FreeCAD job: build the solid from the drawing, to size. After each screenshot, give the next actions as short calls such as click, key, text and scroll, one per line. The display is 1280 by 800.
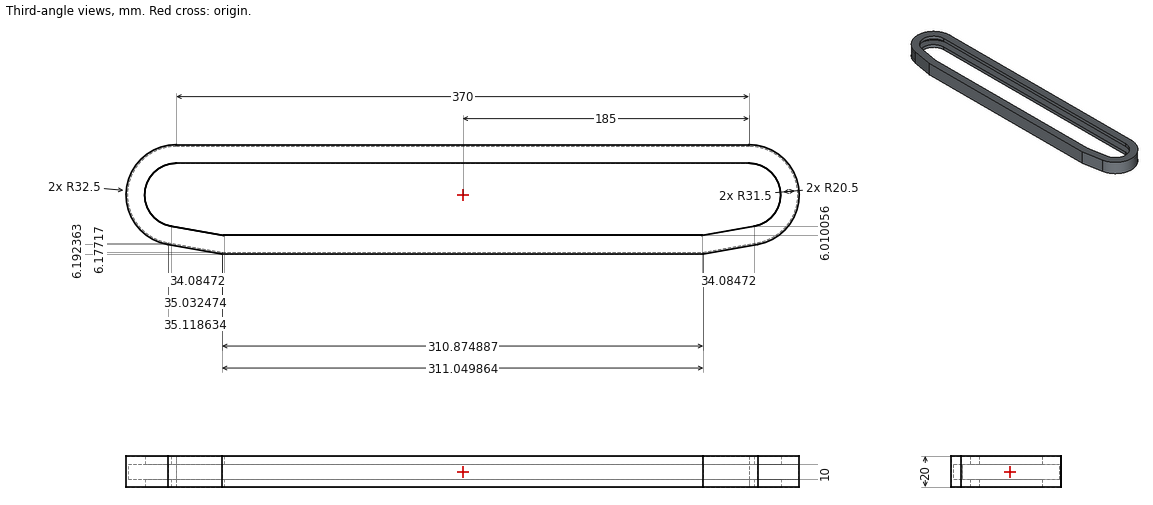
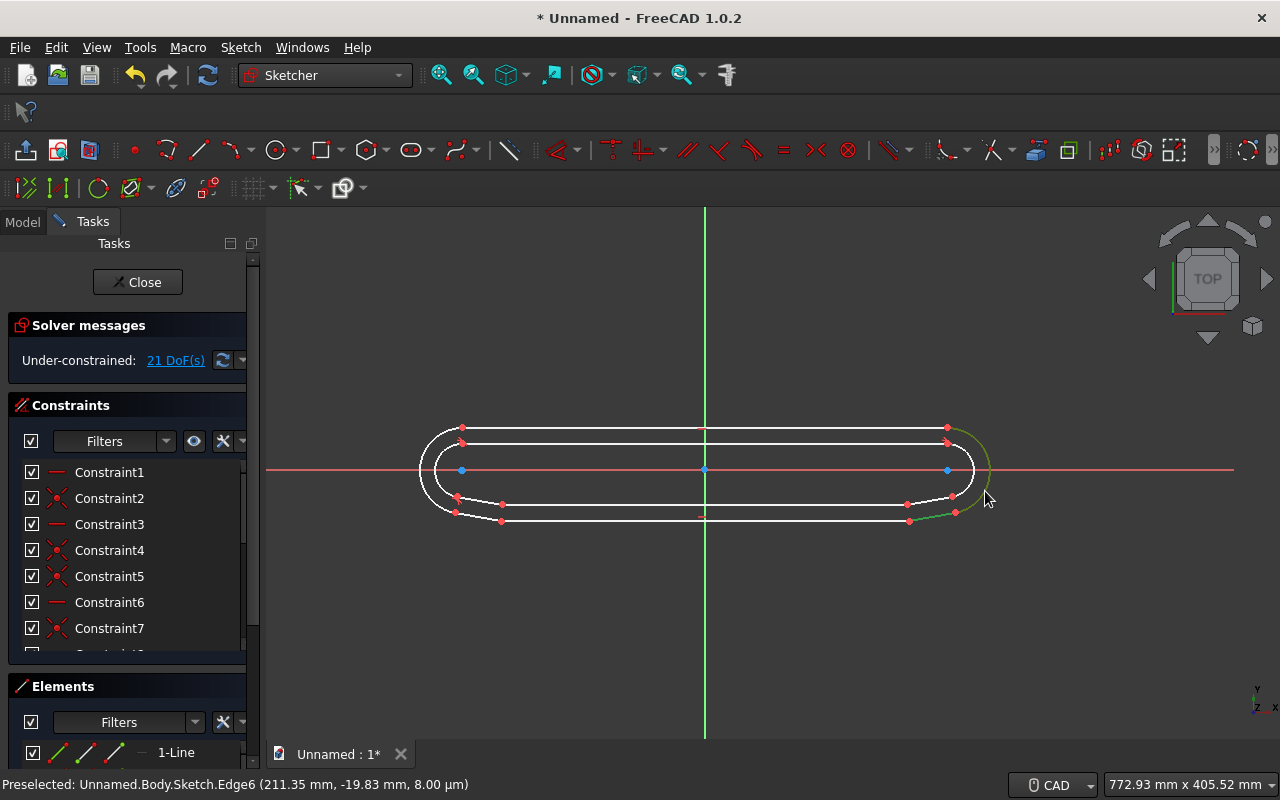
key(t)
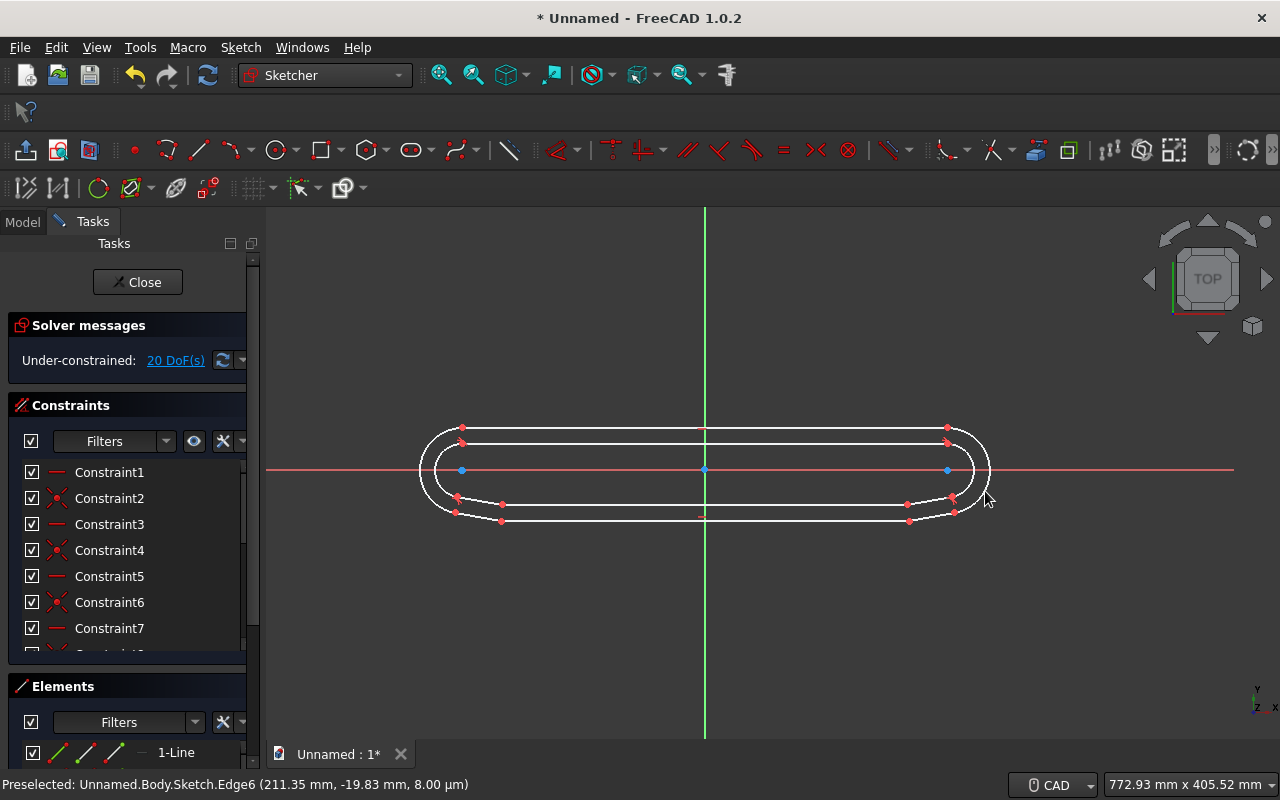
click(607, 444)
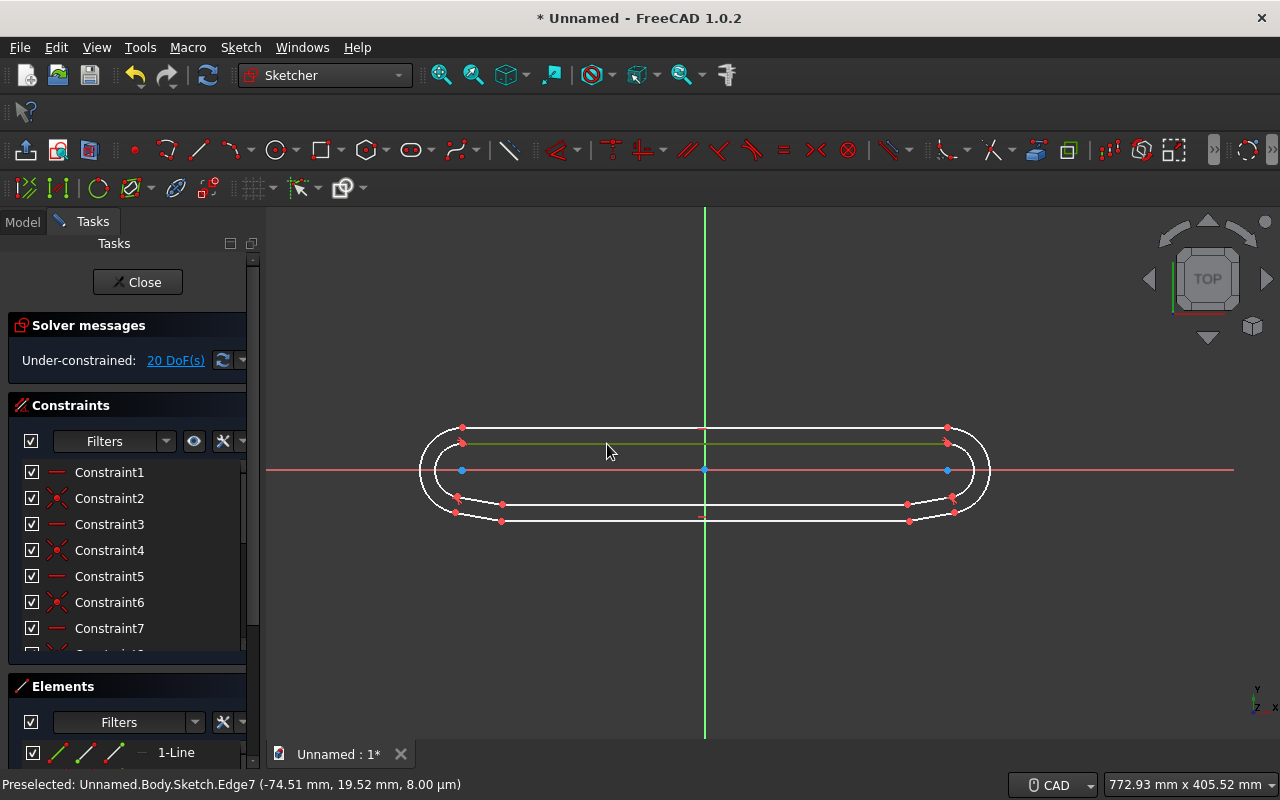
click(971, 484)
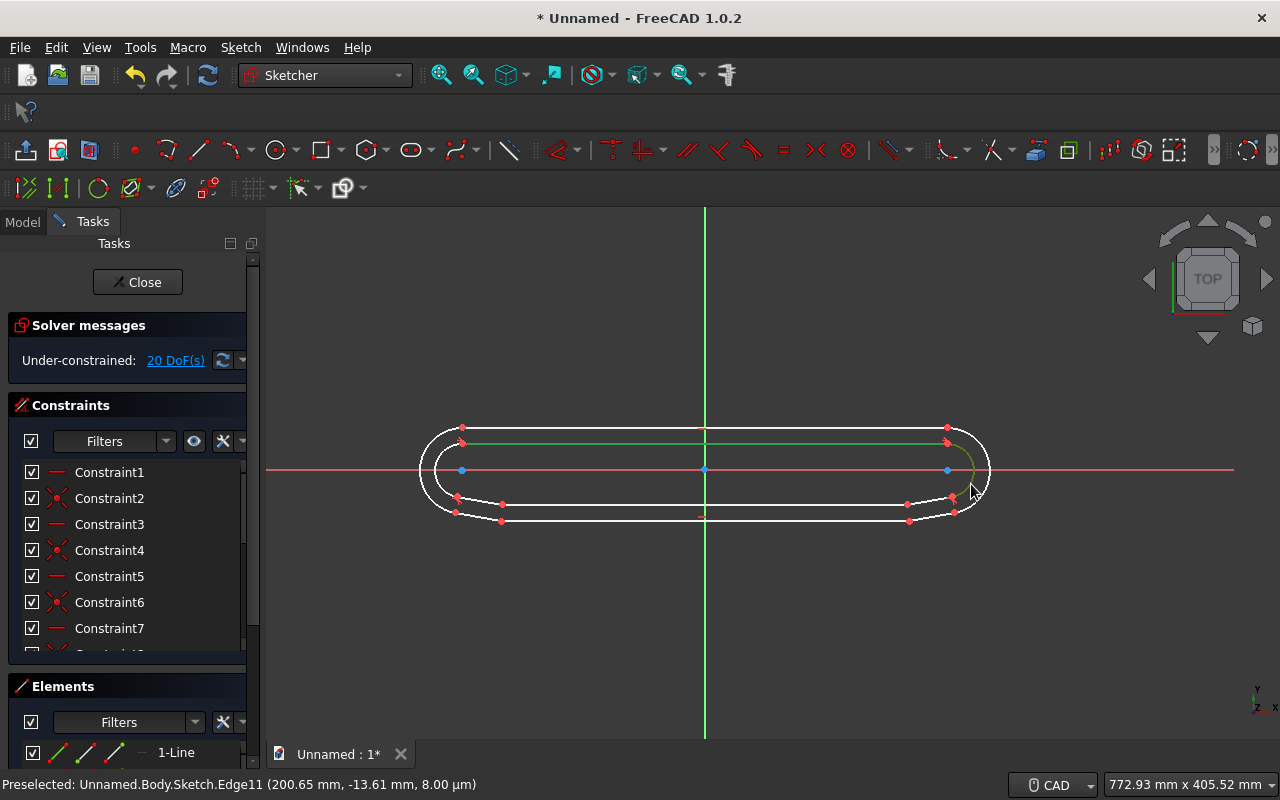
key(t)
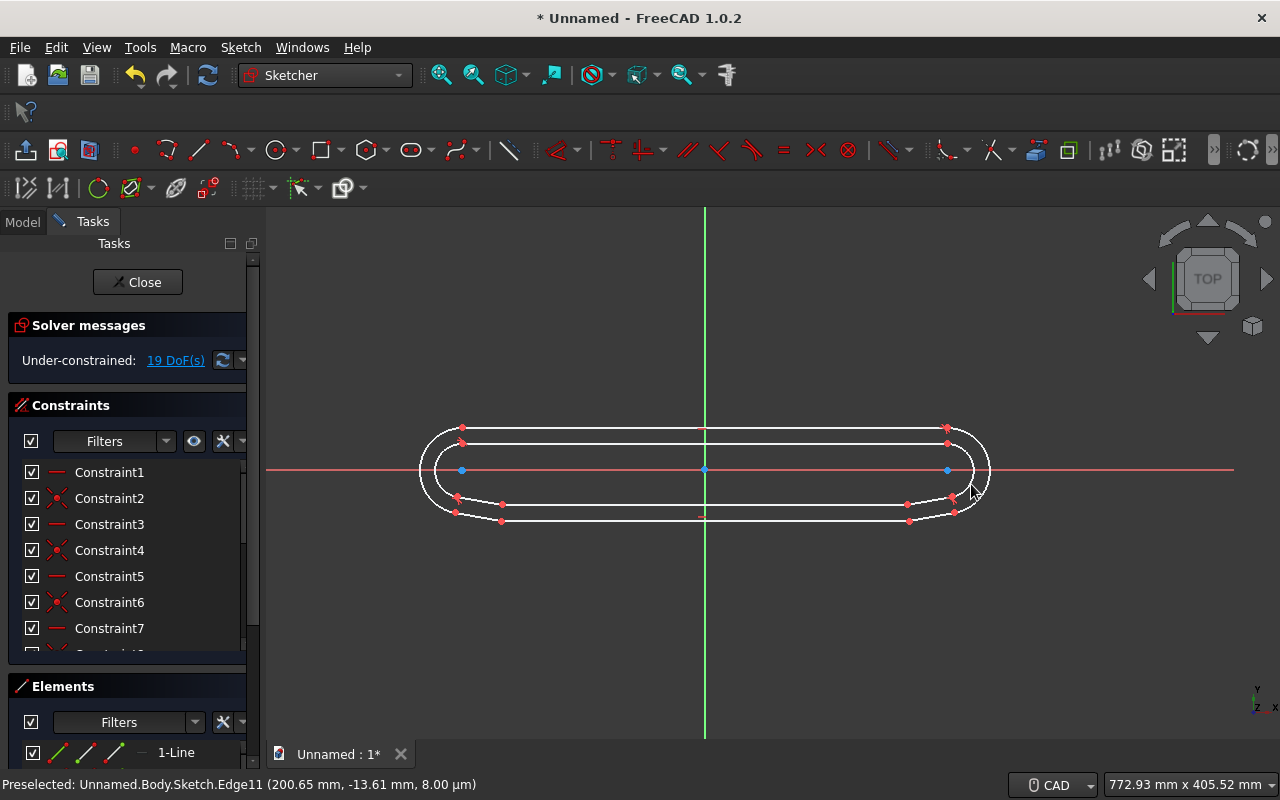
click(607, 444)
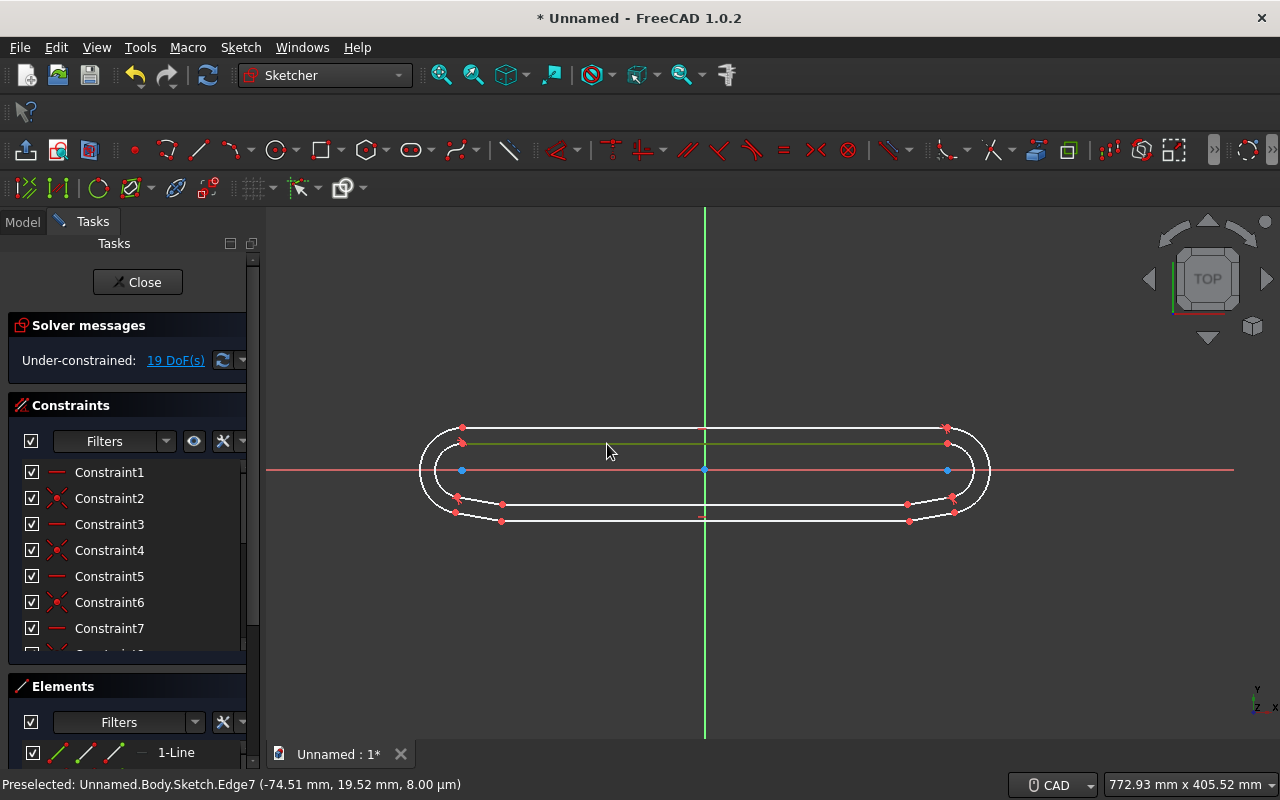
click(441, 454)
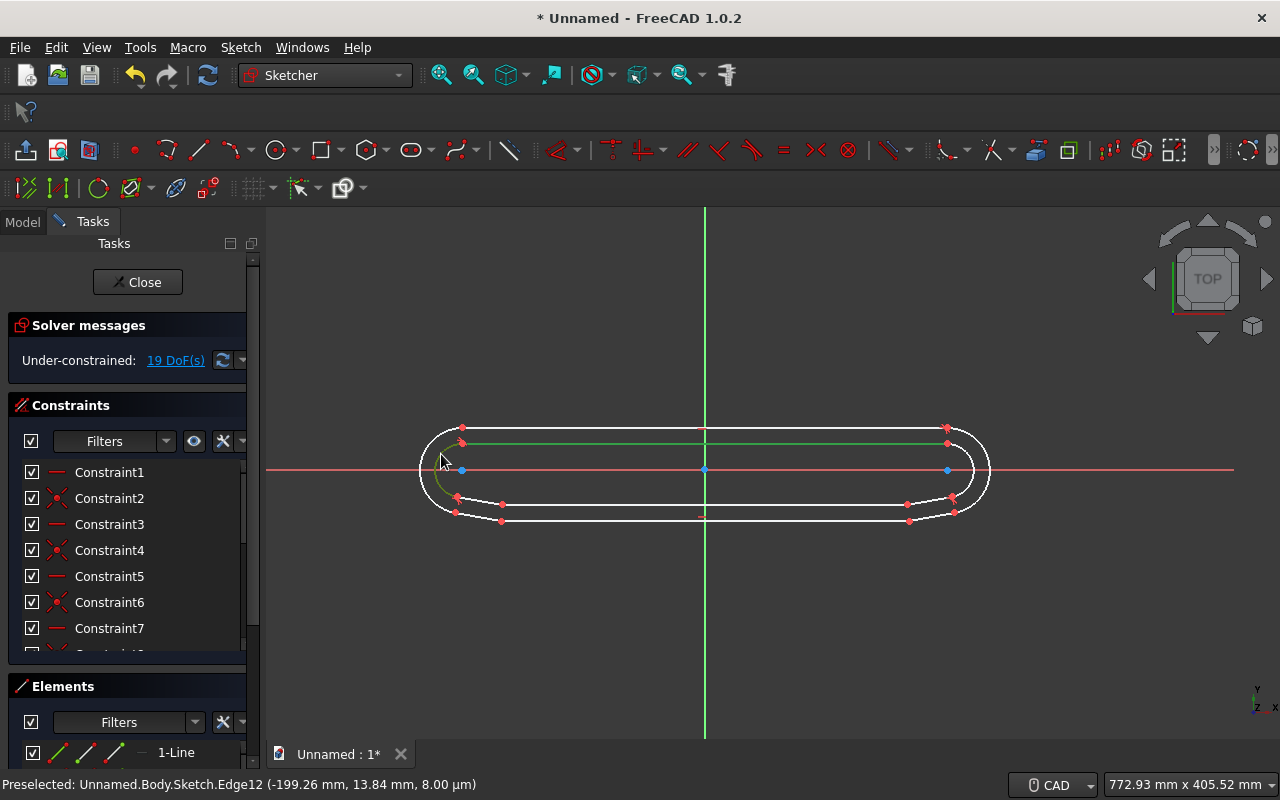
click(752, 150)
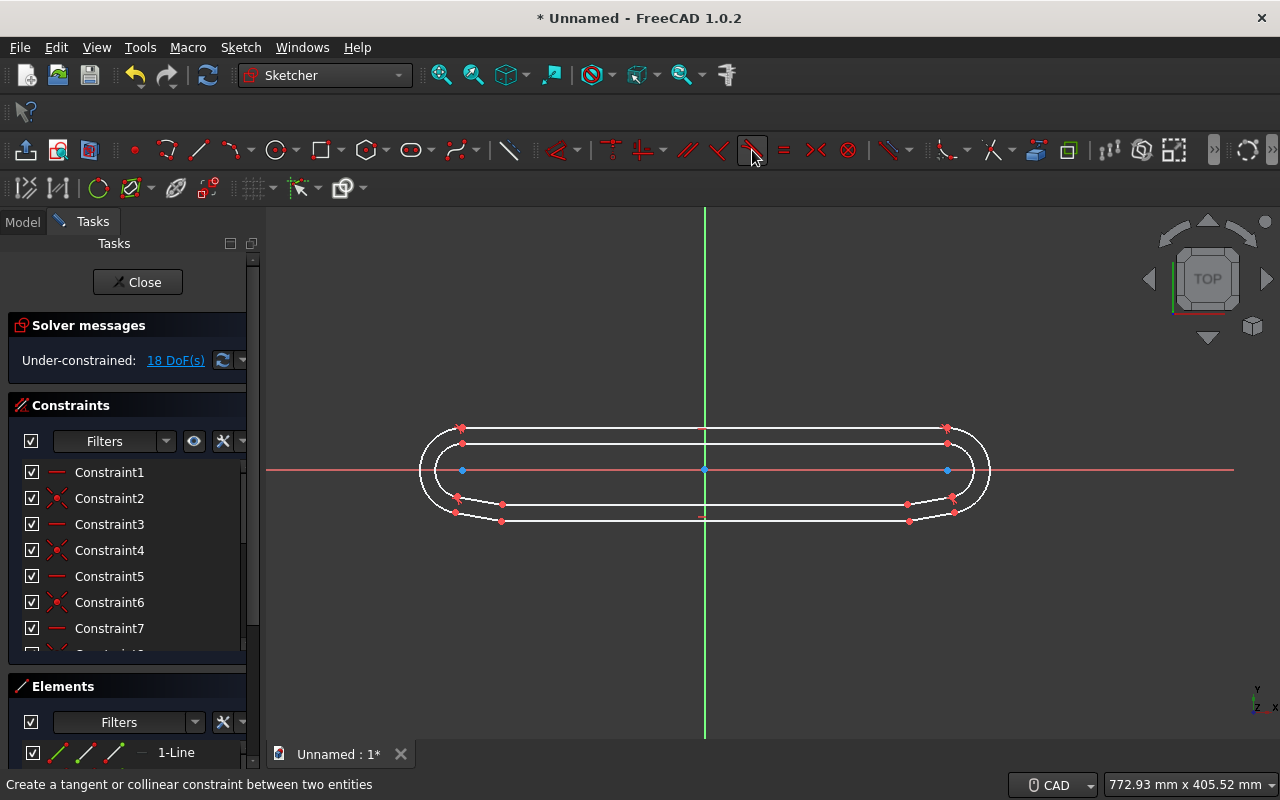
click(938, 499)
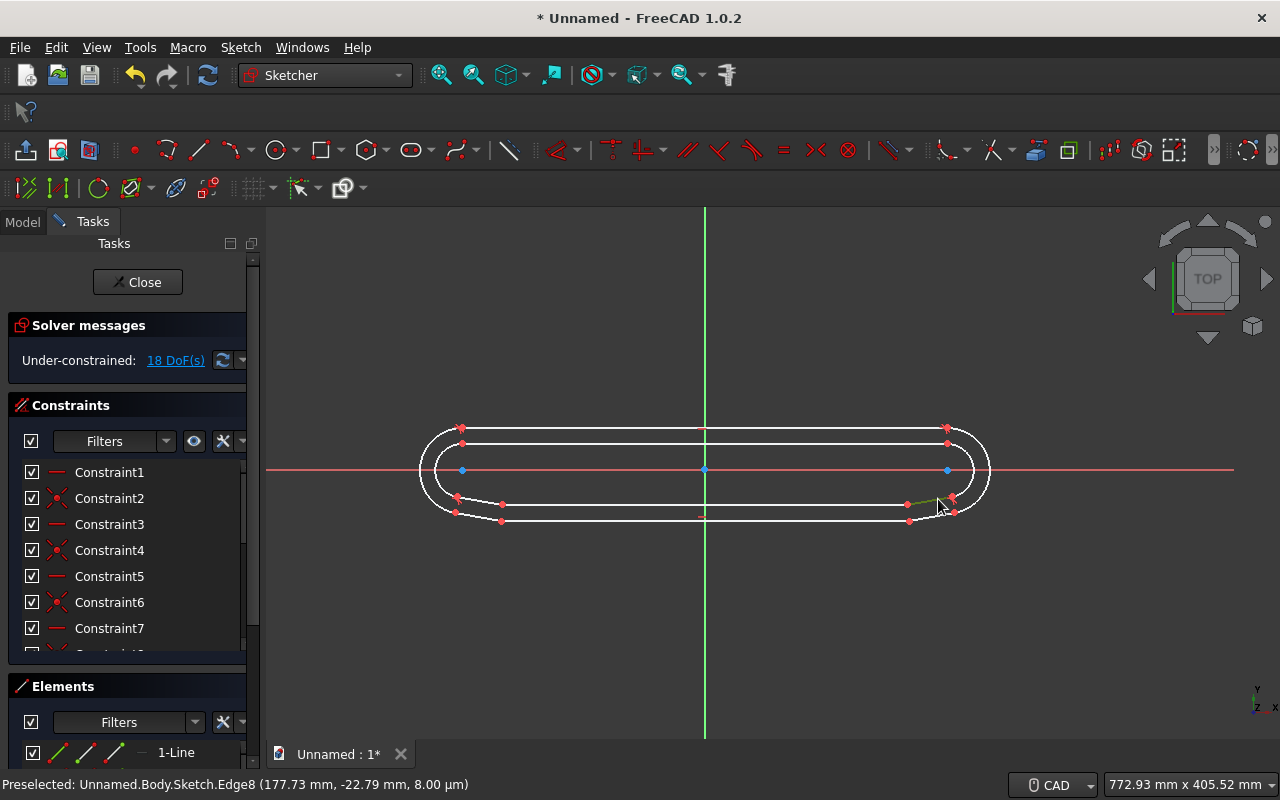
click(971, 483)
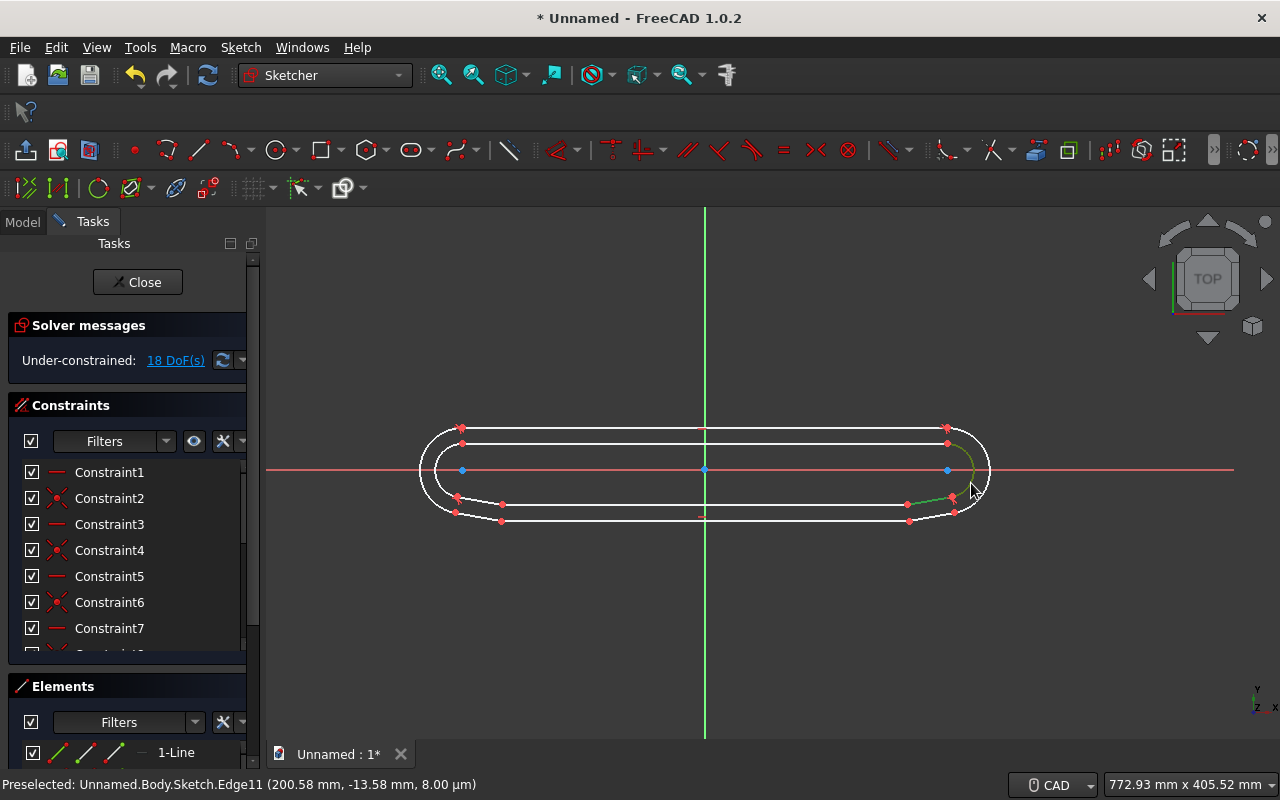
key(t)